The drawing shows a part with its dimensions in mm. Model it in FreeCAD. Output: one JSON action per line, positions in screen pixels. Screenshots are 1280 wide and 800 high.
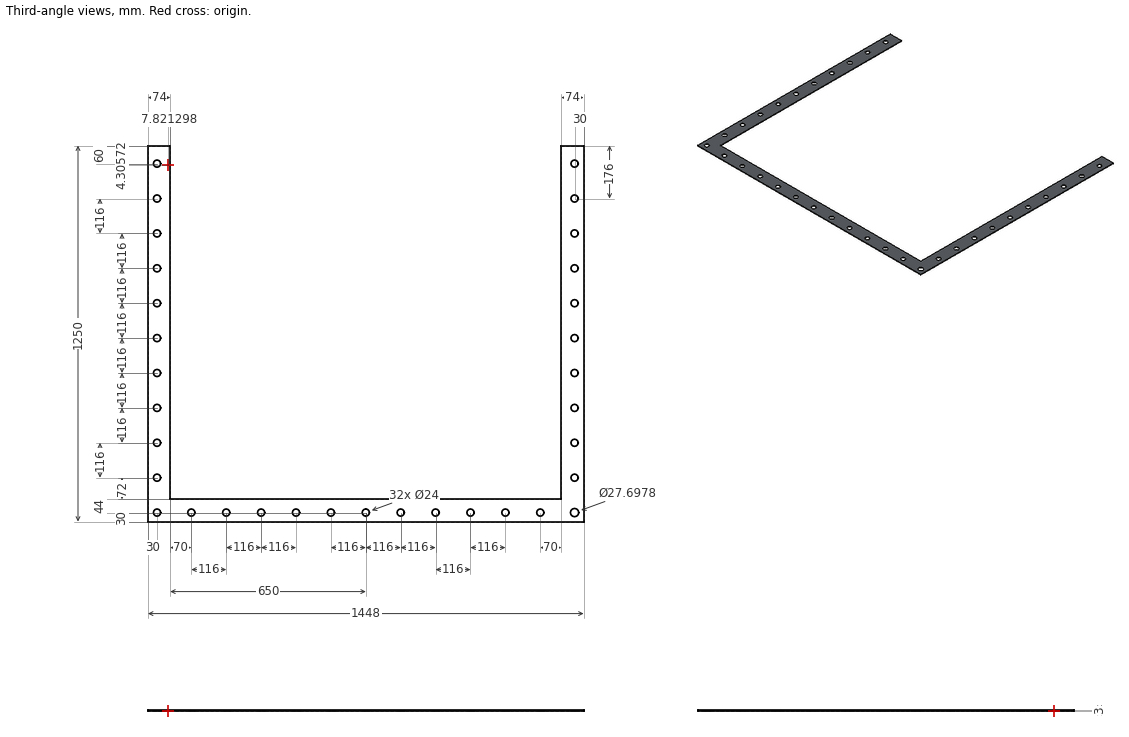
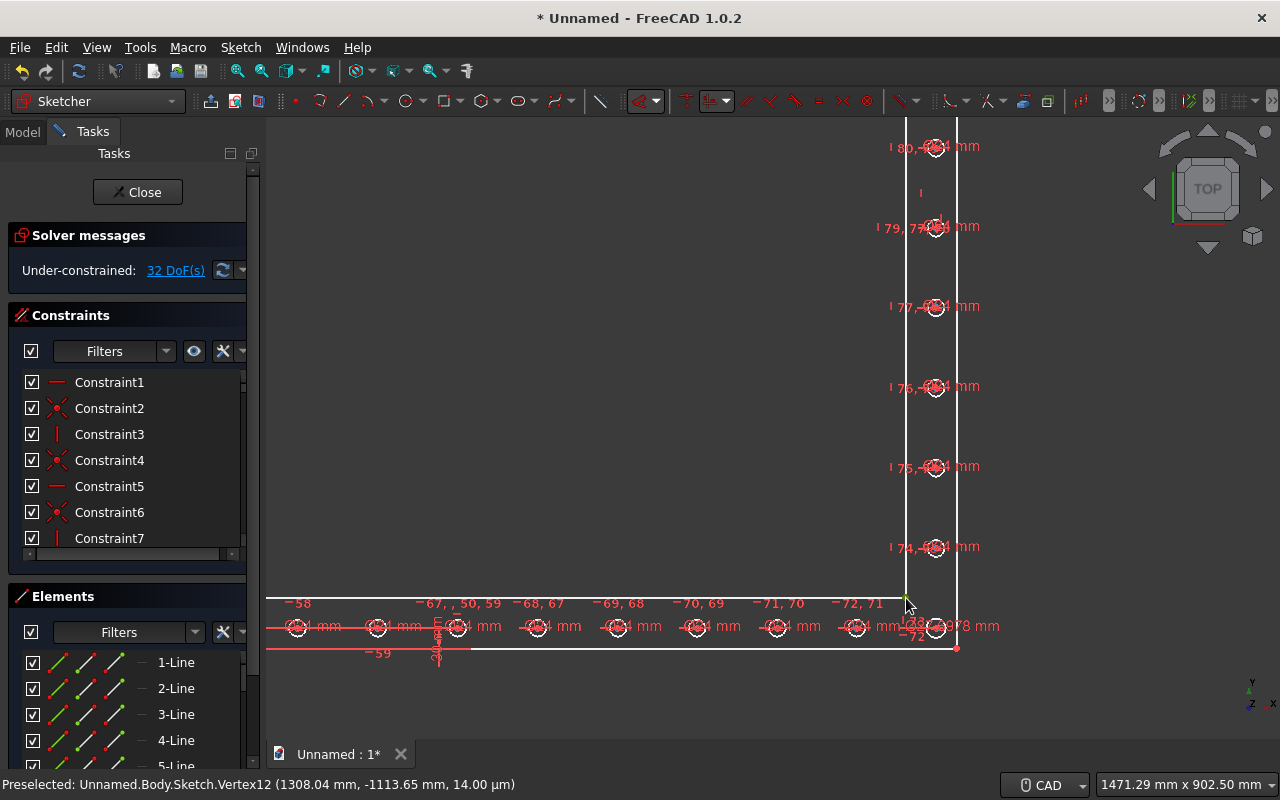
{"action": "left_click", "coordinate": [857, 628]}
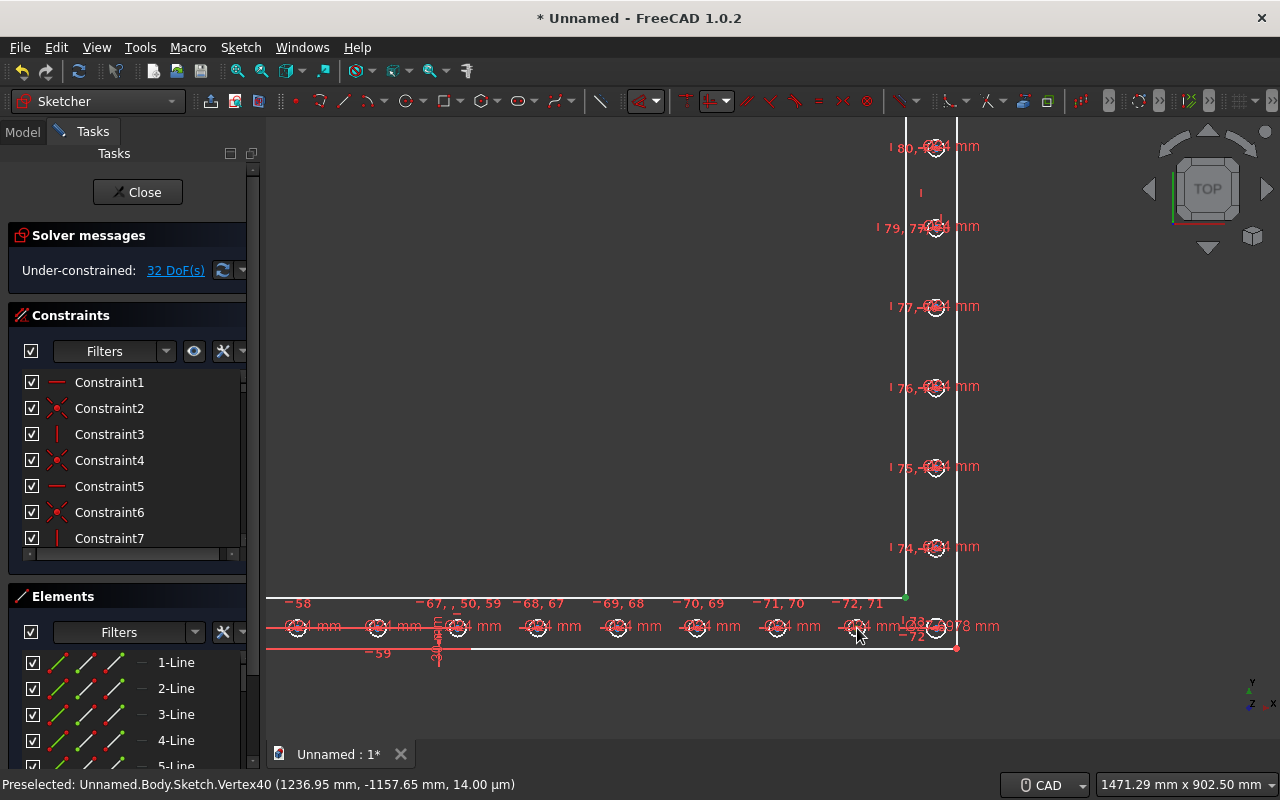
{"action": "key", "text": "l"}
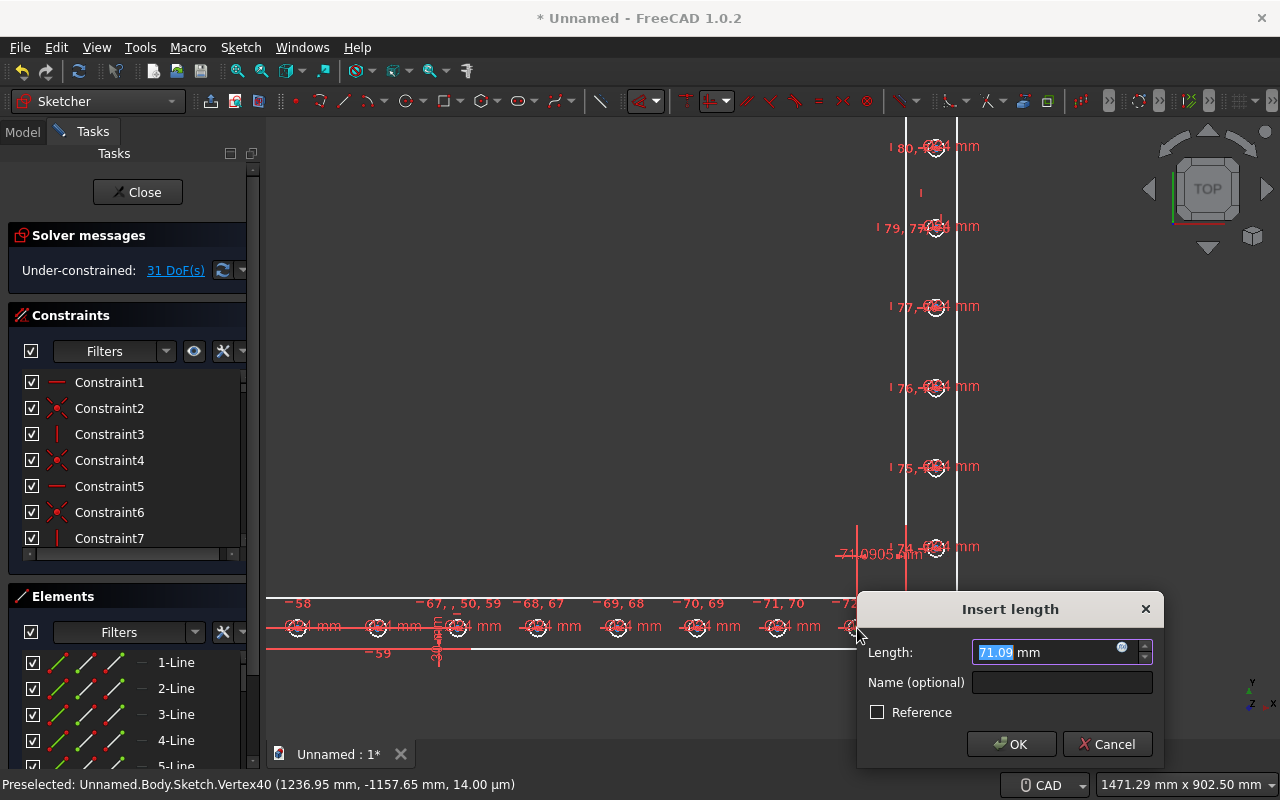
{"action": "type", "text": "70"}
{"action": "key", "text": "Return"}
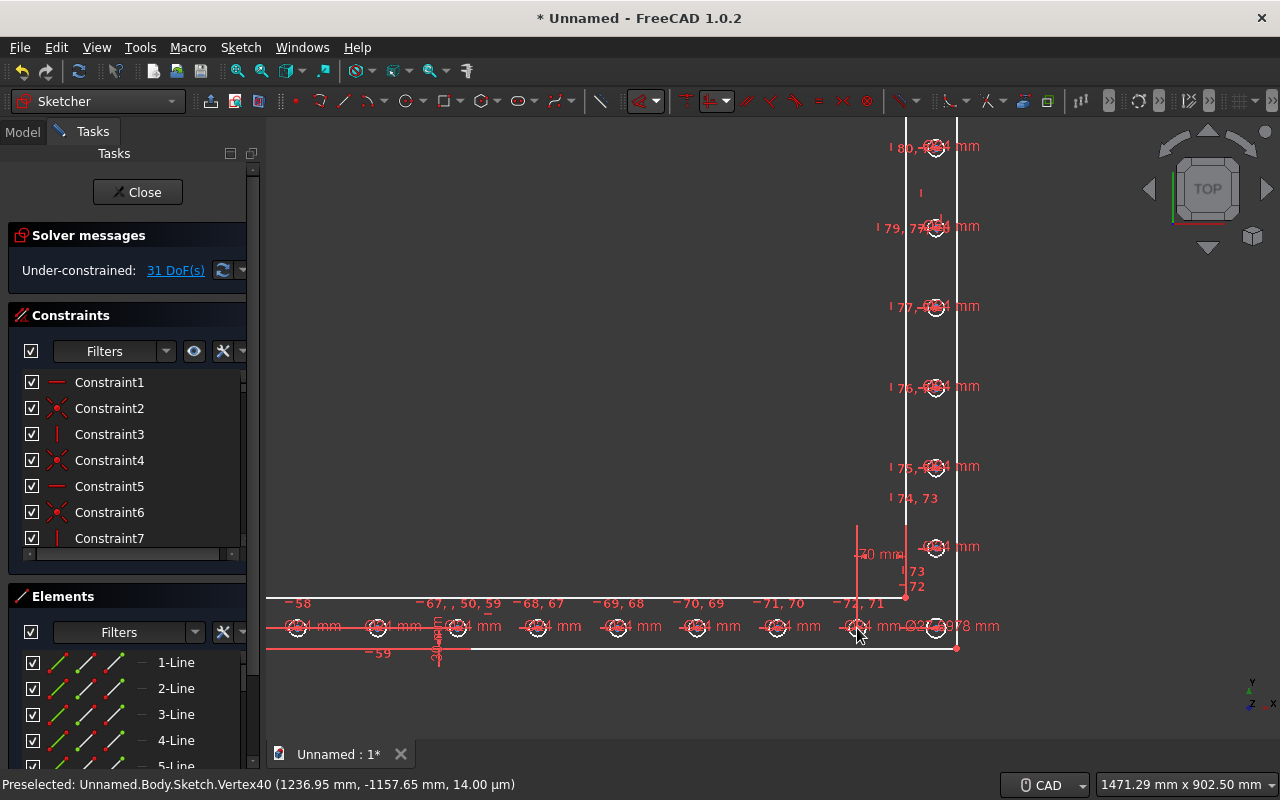
{"action": "left_click", "coordinate": [906, 598]}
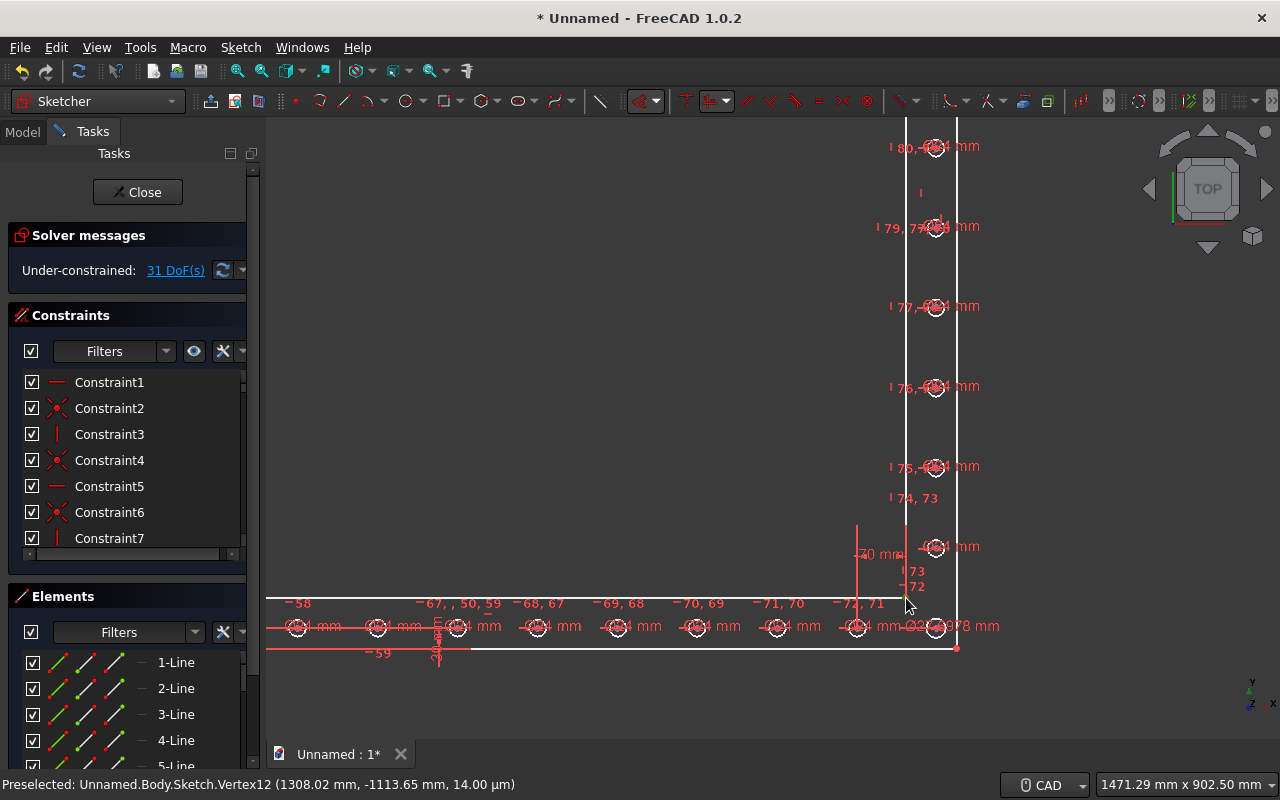
{"action": "left_click", "coordinate": [936, 549]}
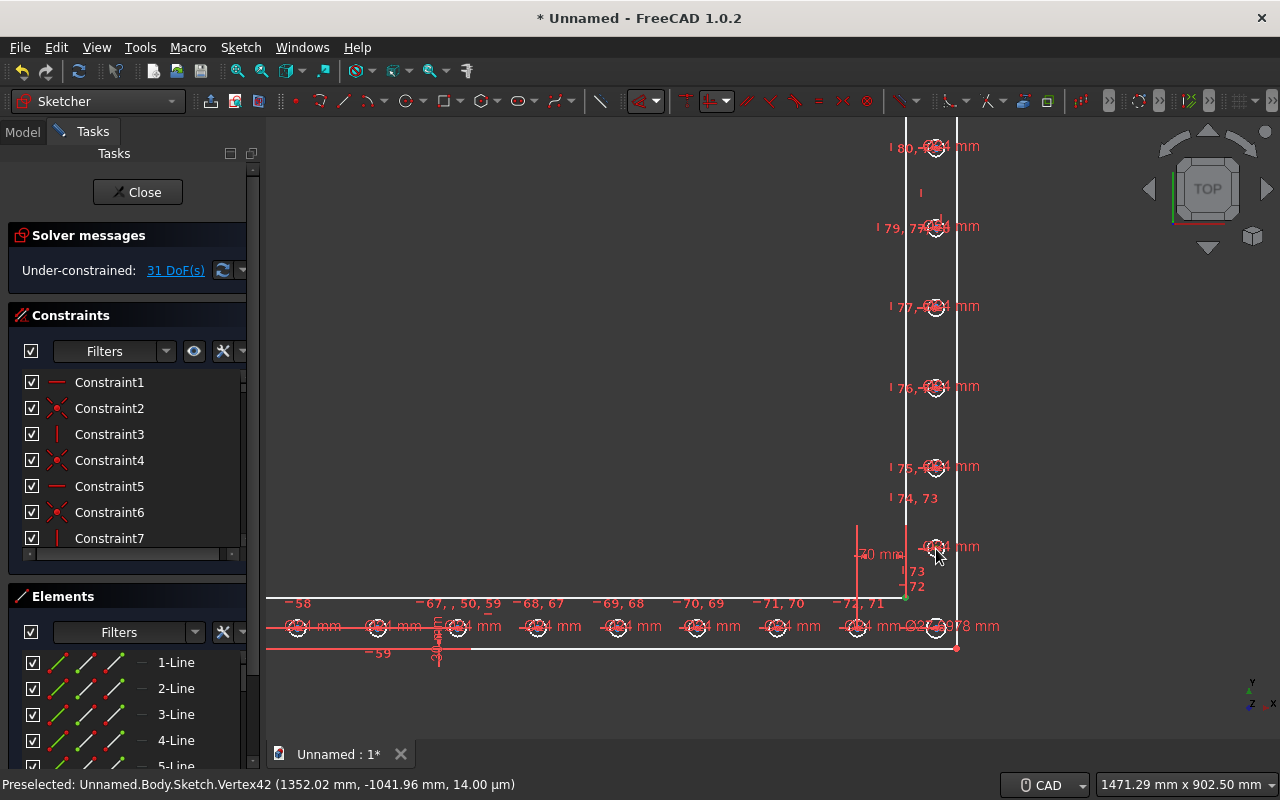
{"action": "key", "text": "i"}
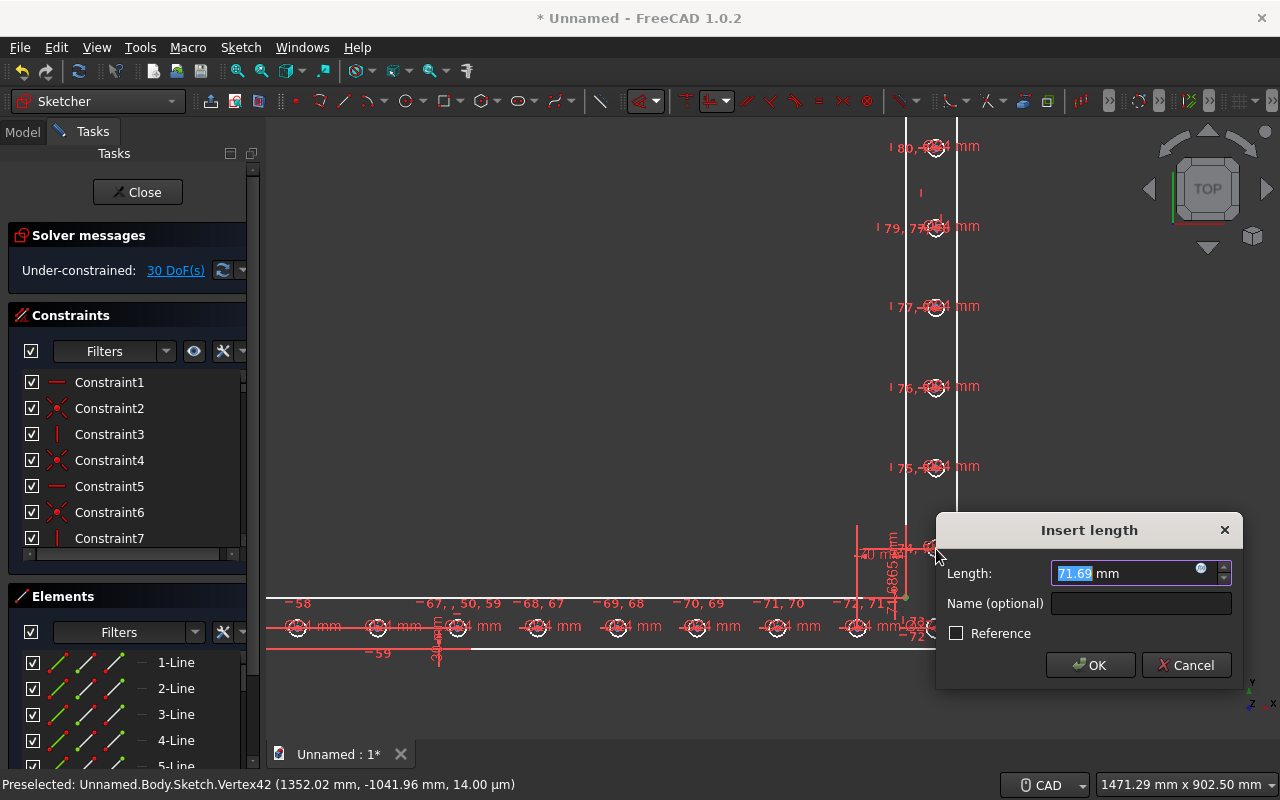
{"action": "type", "text": "72"}
{"action": "key", "text": "Return"}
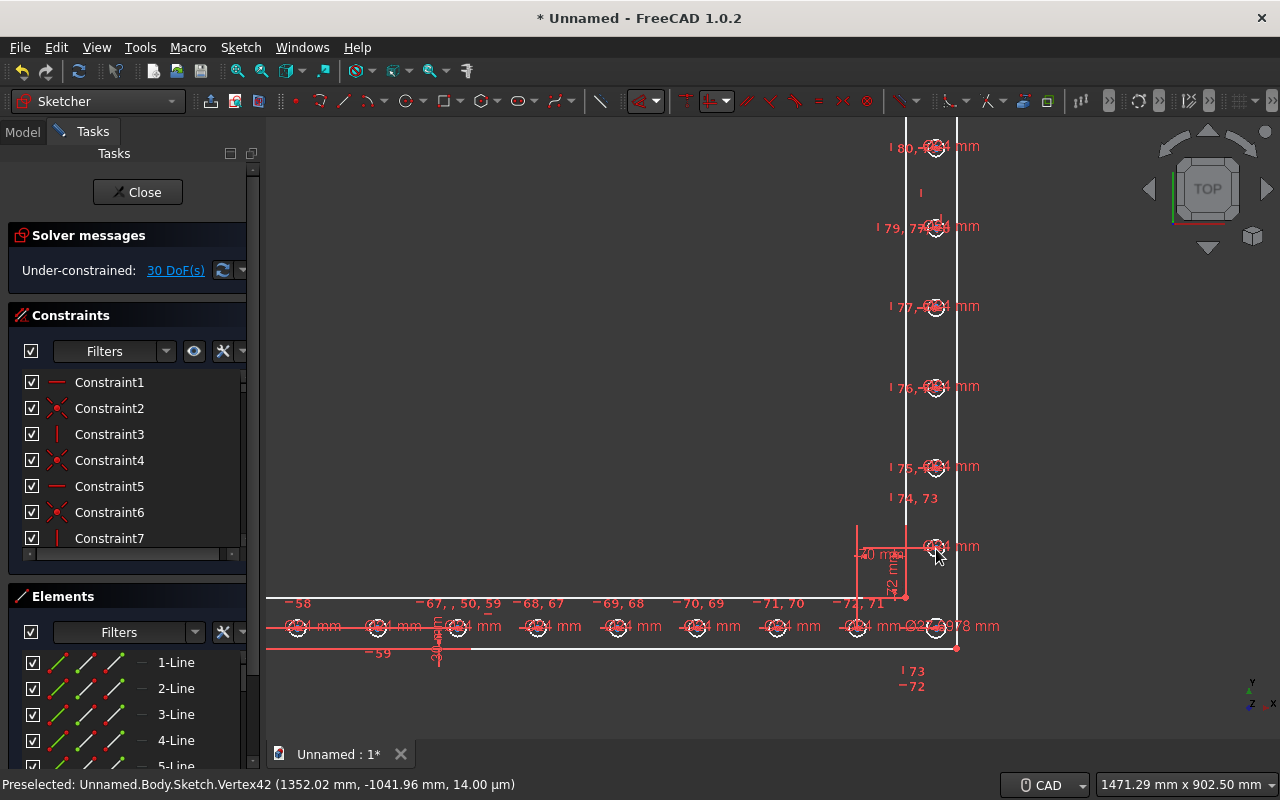
{"action": "scroll", "coordinate": [906, 600], "scroll_direction": "down", "scroll_amount": 4}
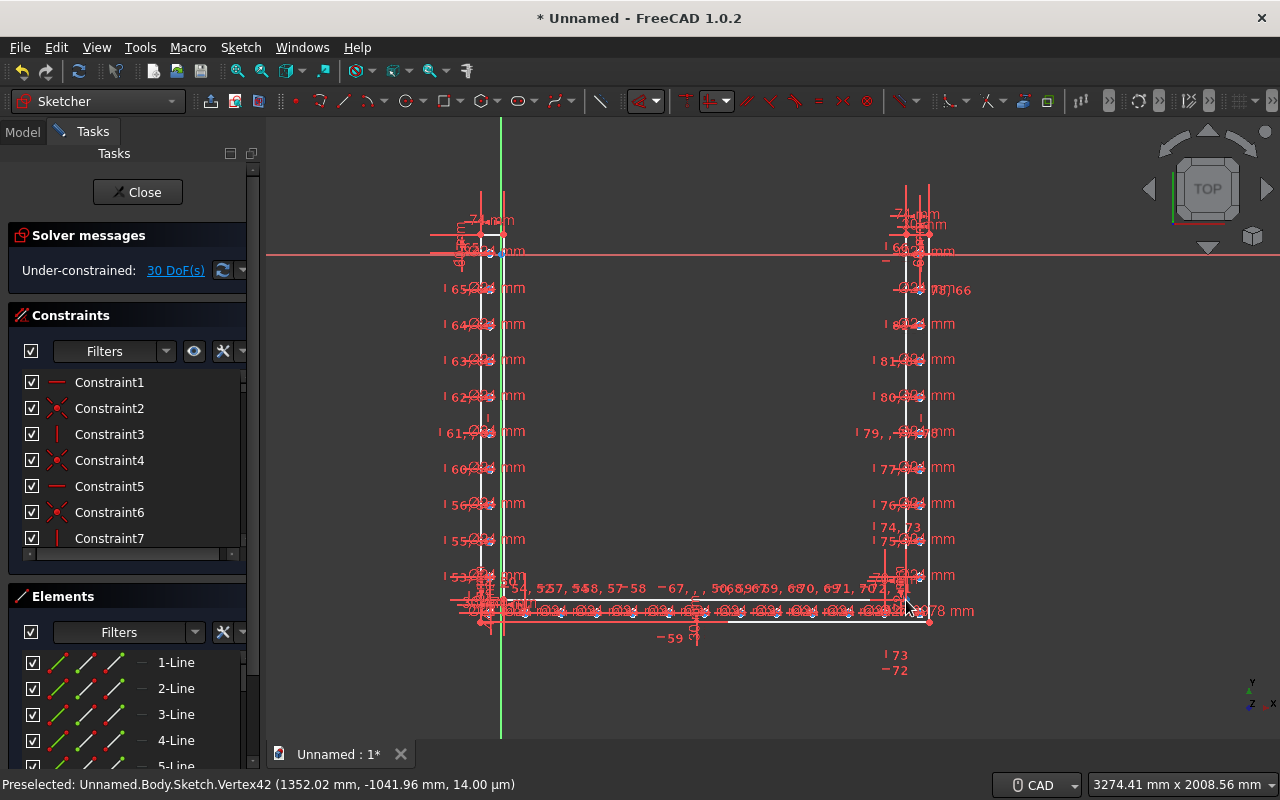
{"action": "scroll", "coordinate": [481, 351], "scroll_direction": "up", "scroll_amount": 2}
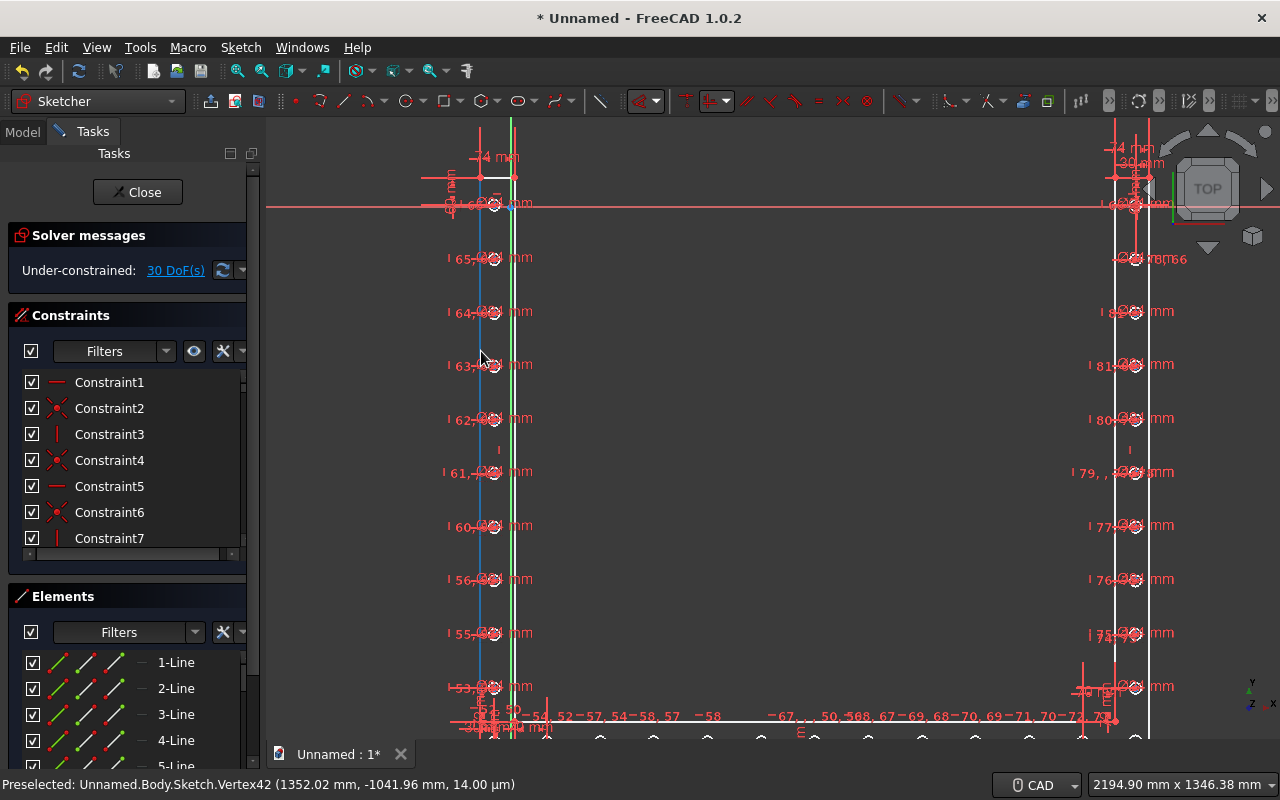
{"action": "left_click", "coordinate": [480, 351]}